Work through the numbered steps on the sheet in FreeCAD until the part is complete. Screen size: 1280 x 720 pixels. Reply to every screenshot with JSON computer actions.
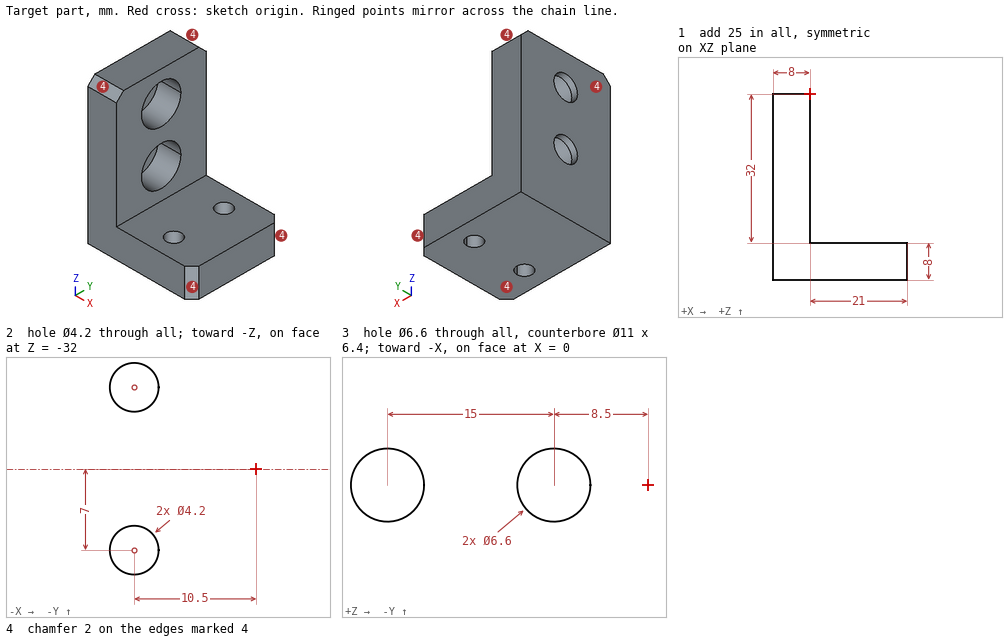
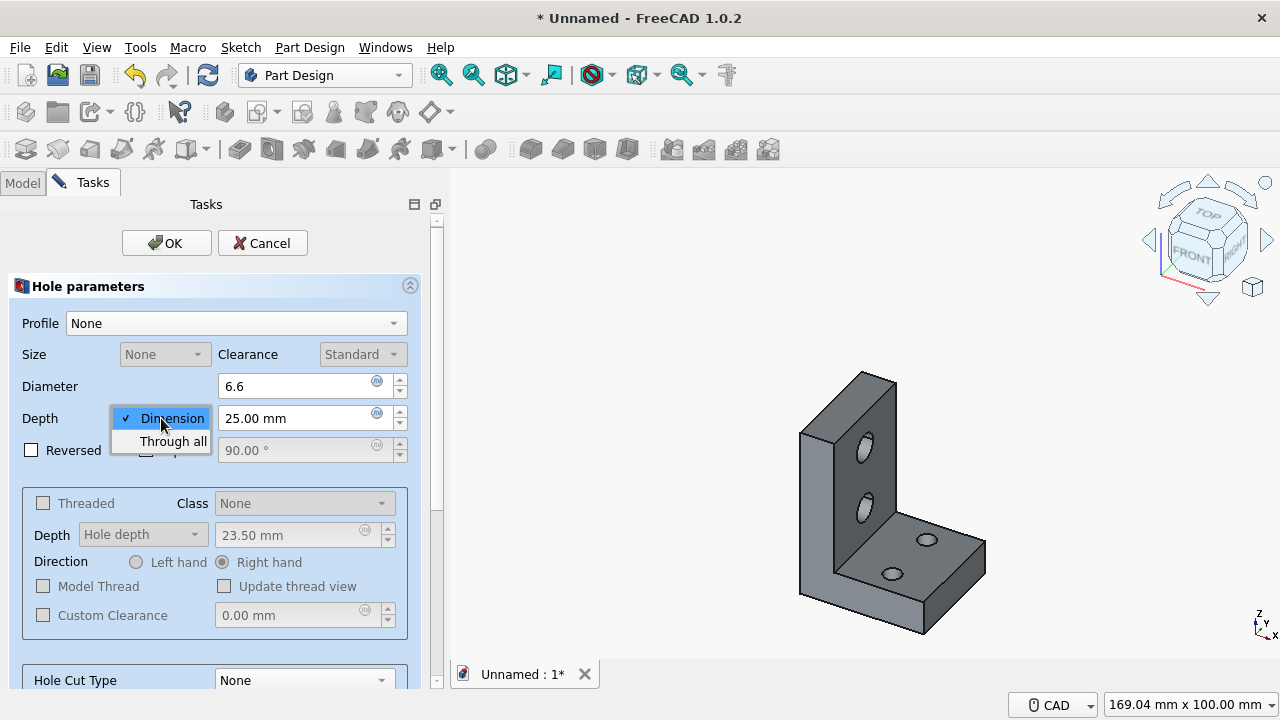
{"action": "left_click", "coordinate": [160, 442]}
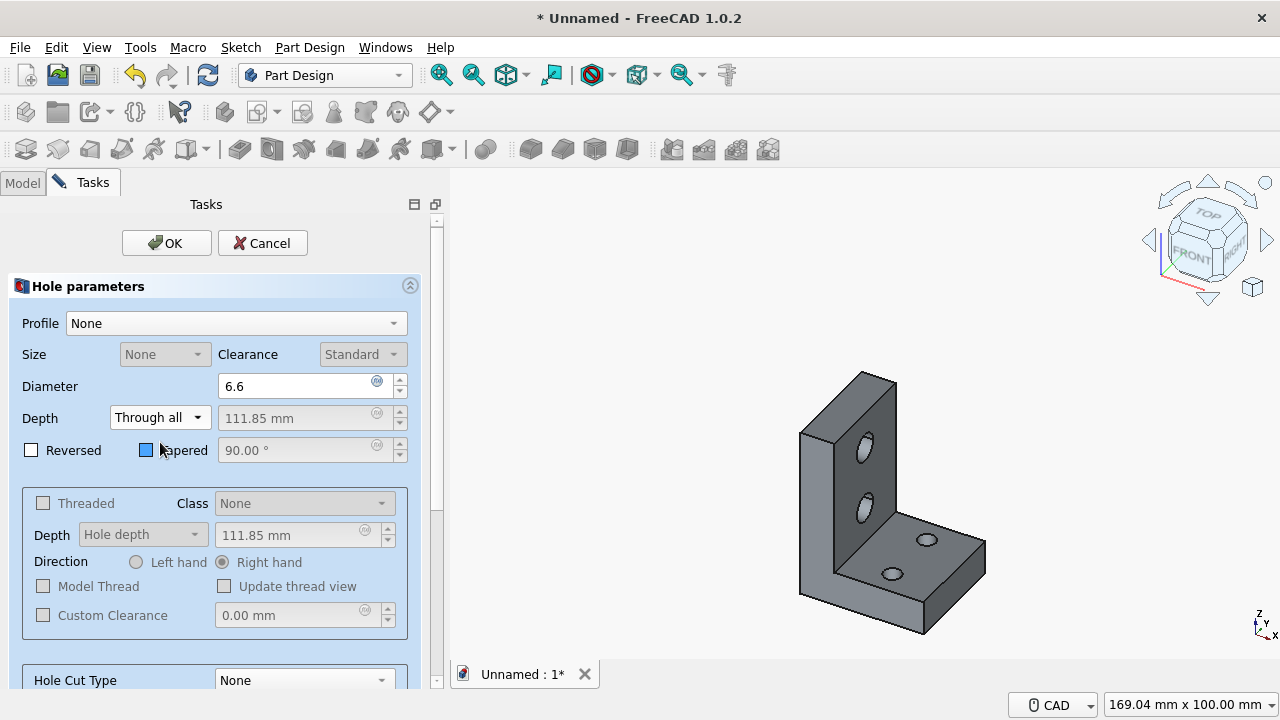
{"action": "scroll", "coordinate": [437, 451], "scroll_direction": "down", "scroll_amount": 2}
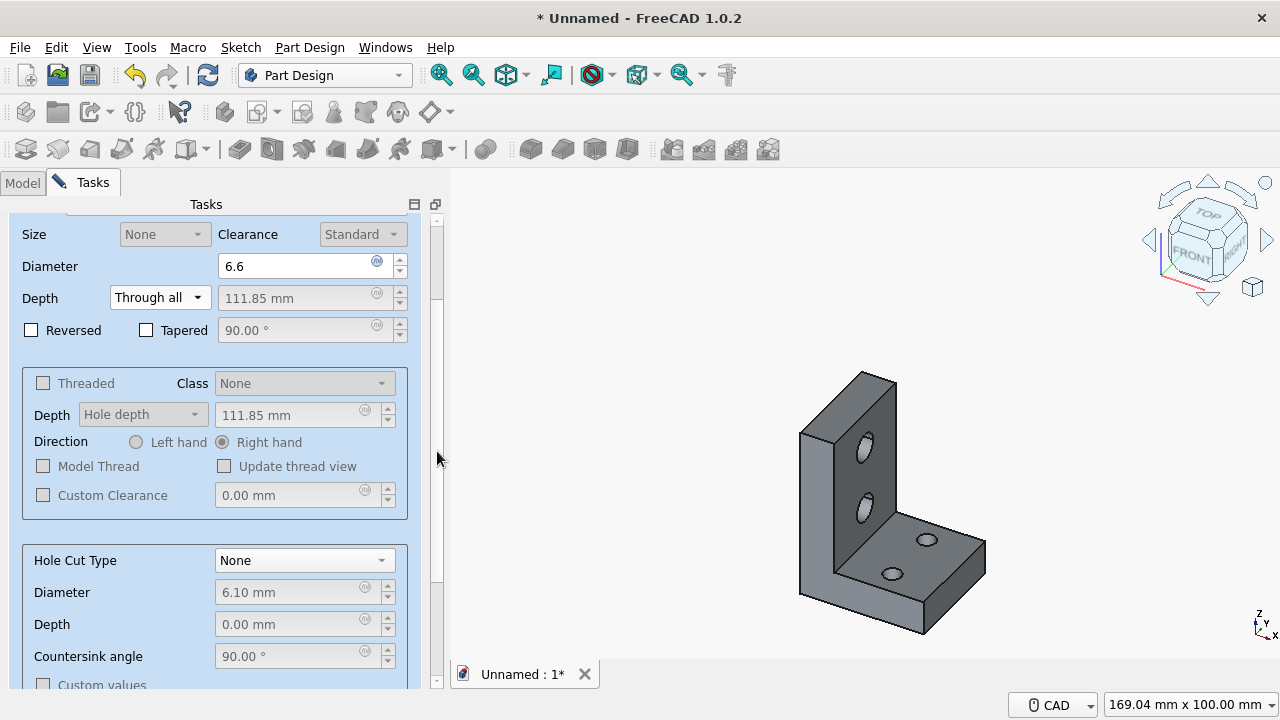
{"action": "left_click", "coordinate": [306, 560]}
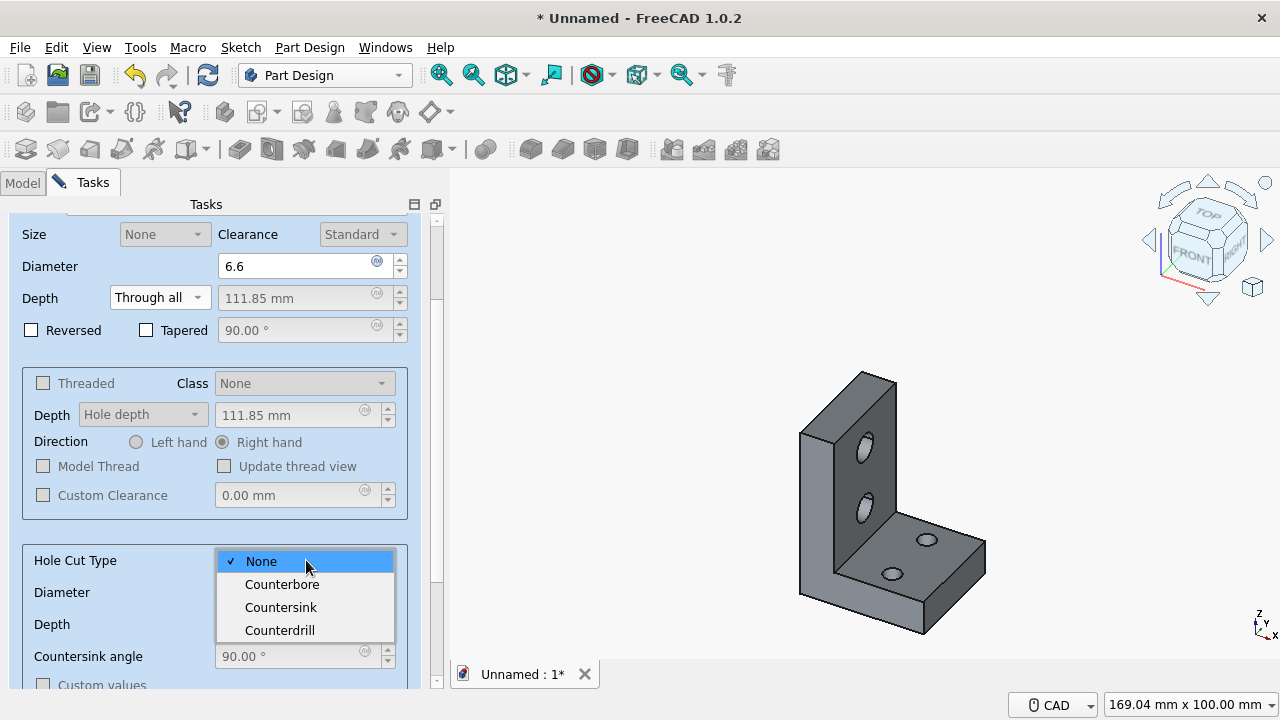
{"action": "left_click", "coordinate": [304, 584]}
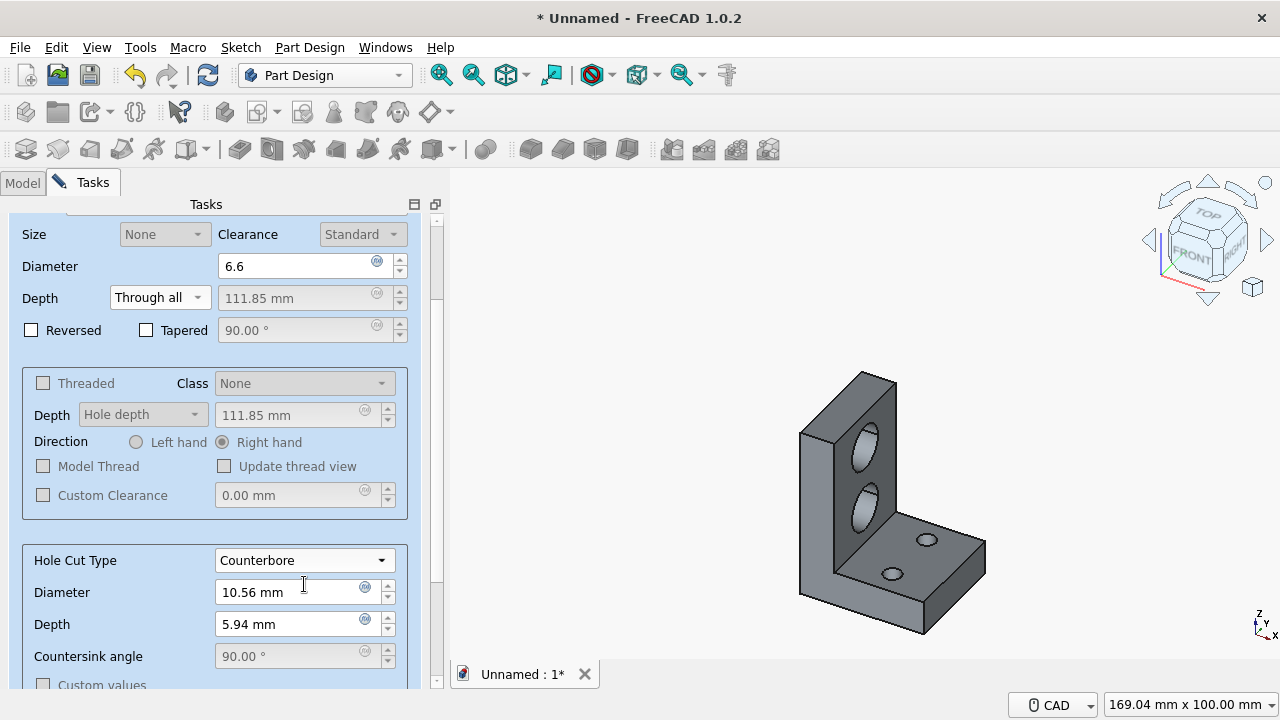
{"action": "triple_click", "coordinate": [298, 592]}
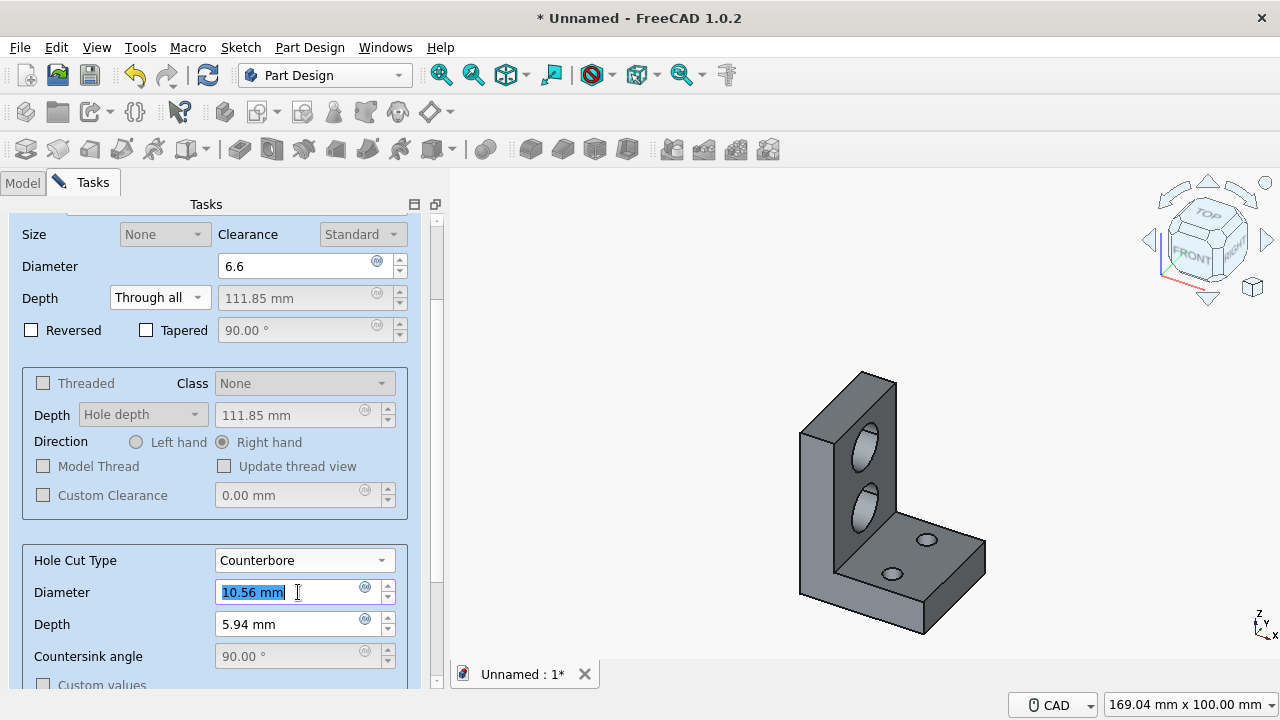
{"action": "type", "text": "11"}
{"action": "key", "text": "Tab"}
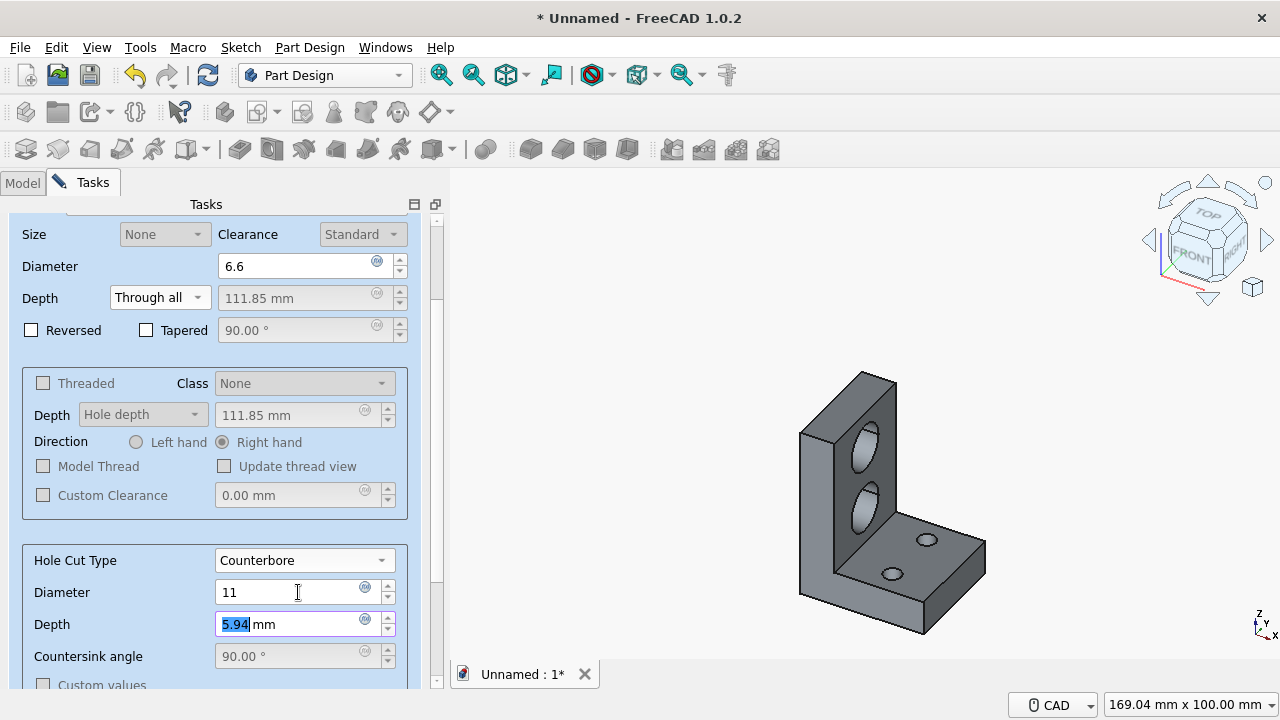
{"action": "type", "text": "6.4"}
{"action": "key", "text": "Tab"}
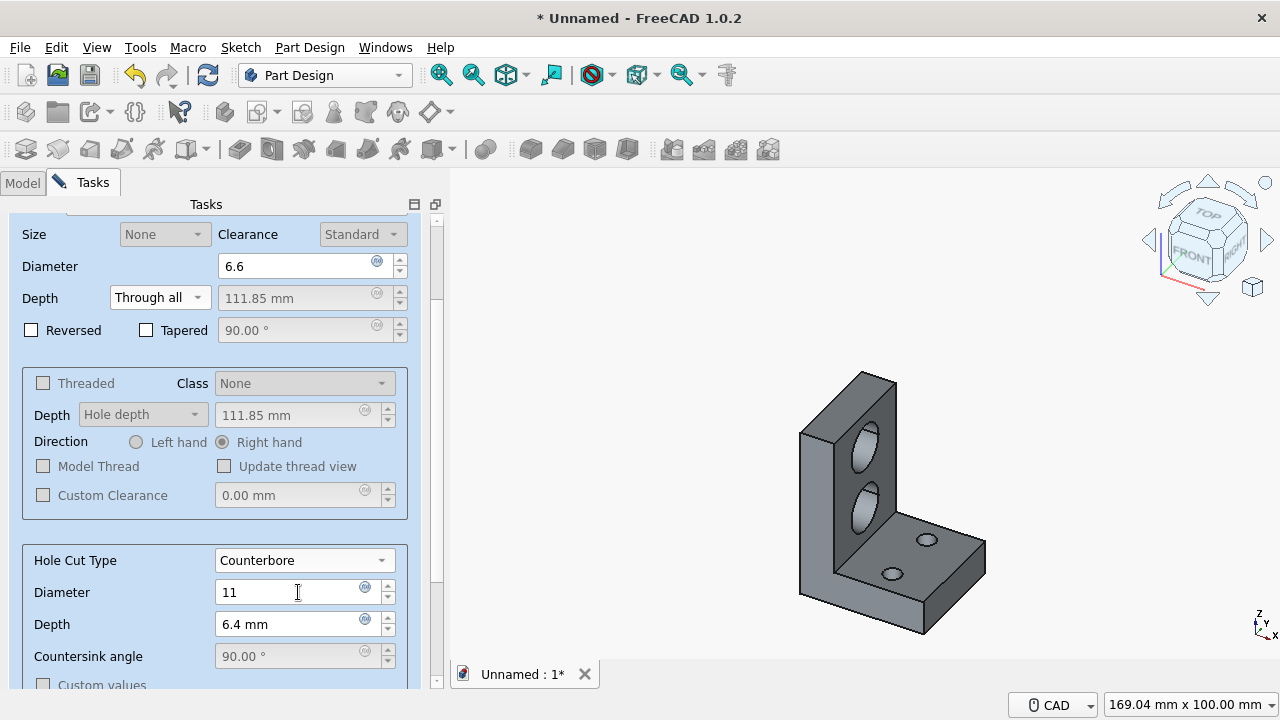
{"action": "scroll", "coordinate": [437, 451], "scroll_direction": "up", "scroll_amount": 3}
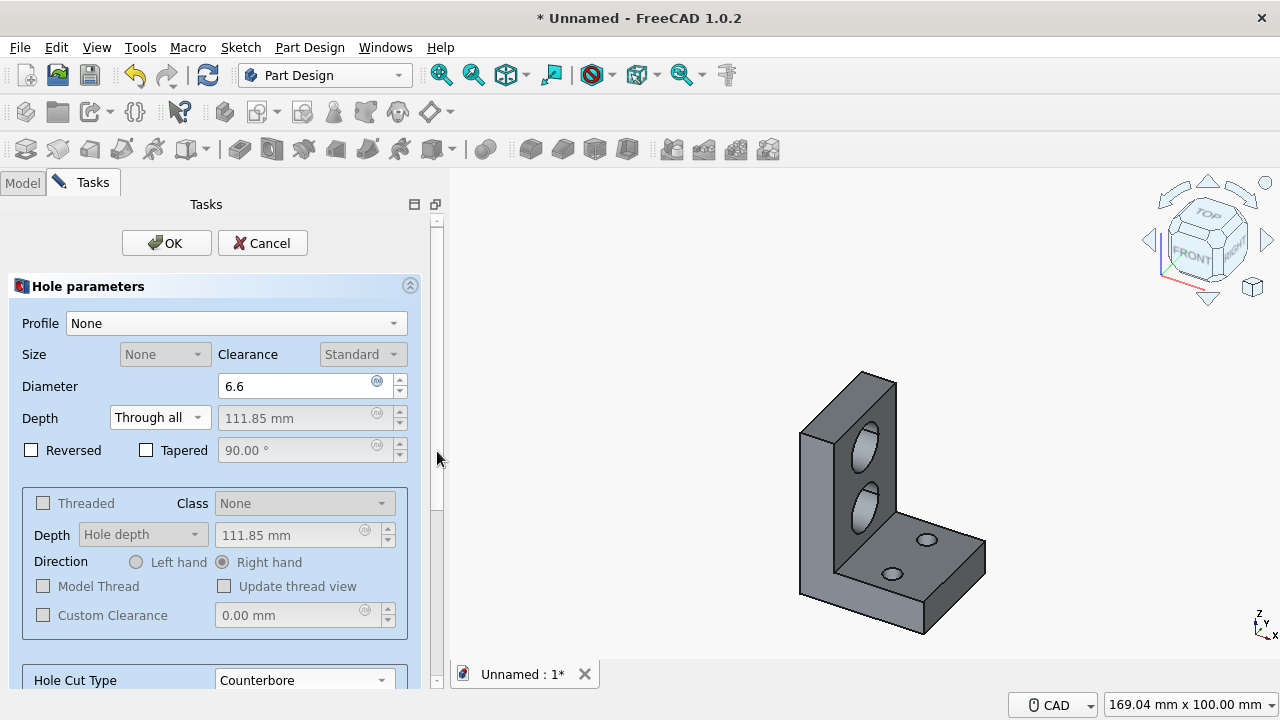
{"action": "left_click", "coordinate": [167, 243]}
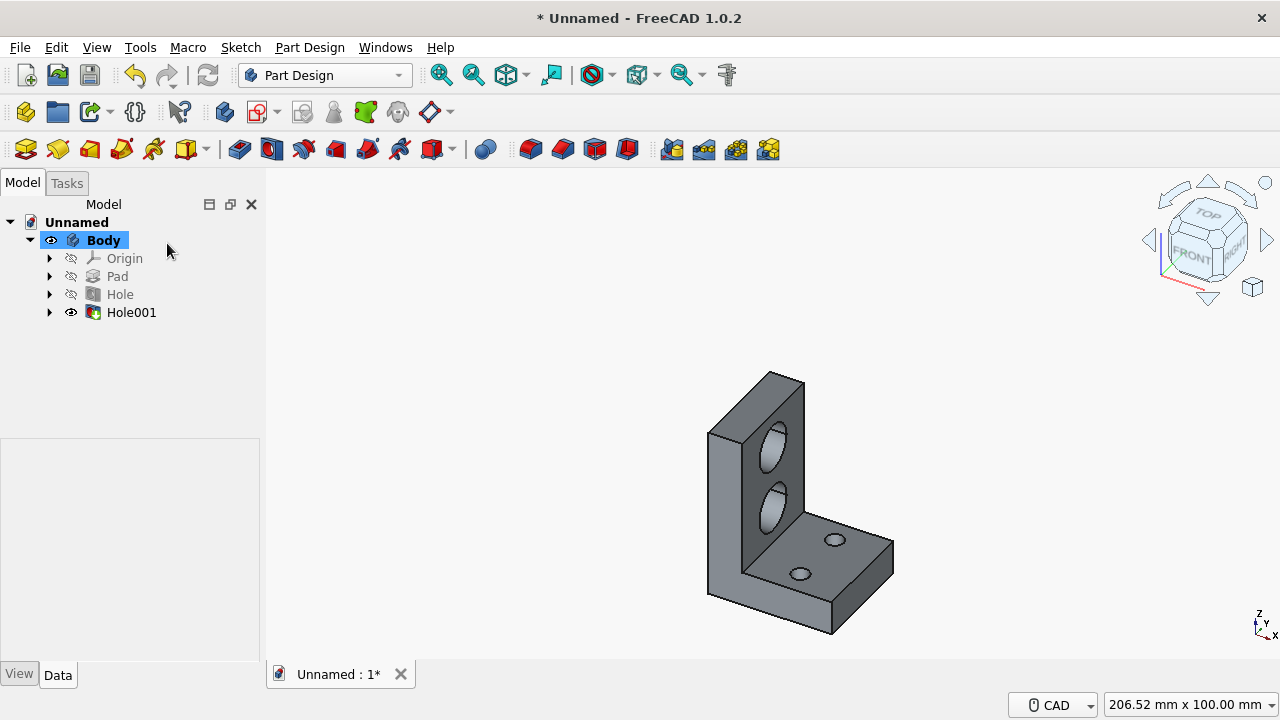
{"action": "left_click", "coordinate": [832, 617]}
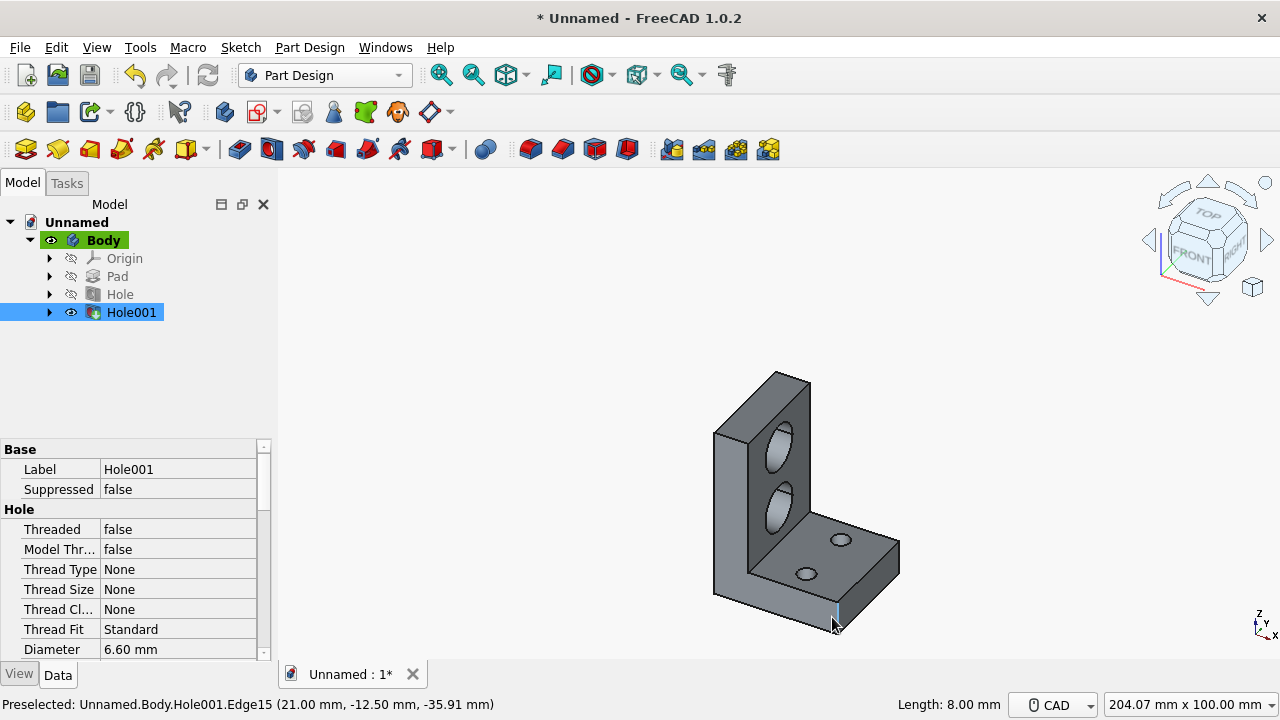
{"action": "left_click", "coordinate": [731, 437], "text": "ctrl"}